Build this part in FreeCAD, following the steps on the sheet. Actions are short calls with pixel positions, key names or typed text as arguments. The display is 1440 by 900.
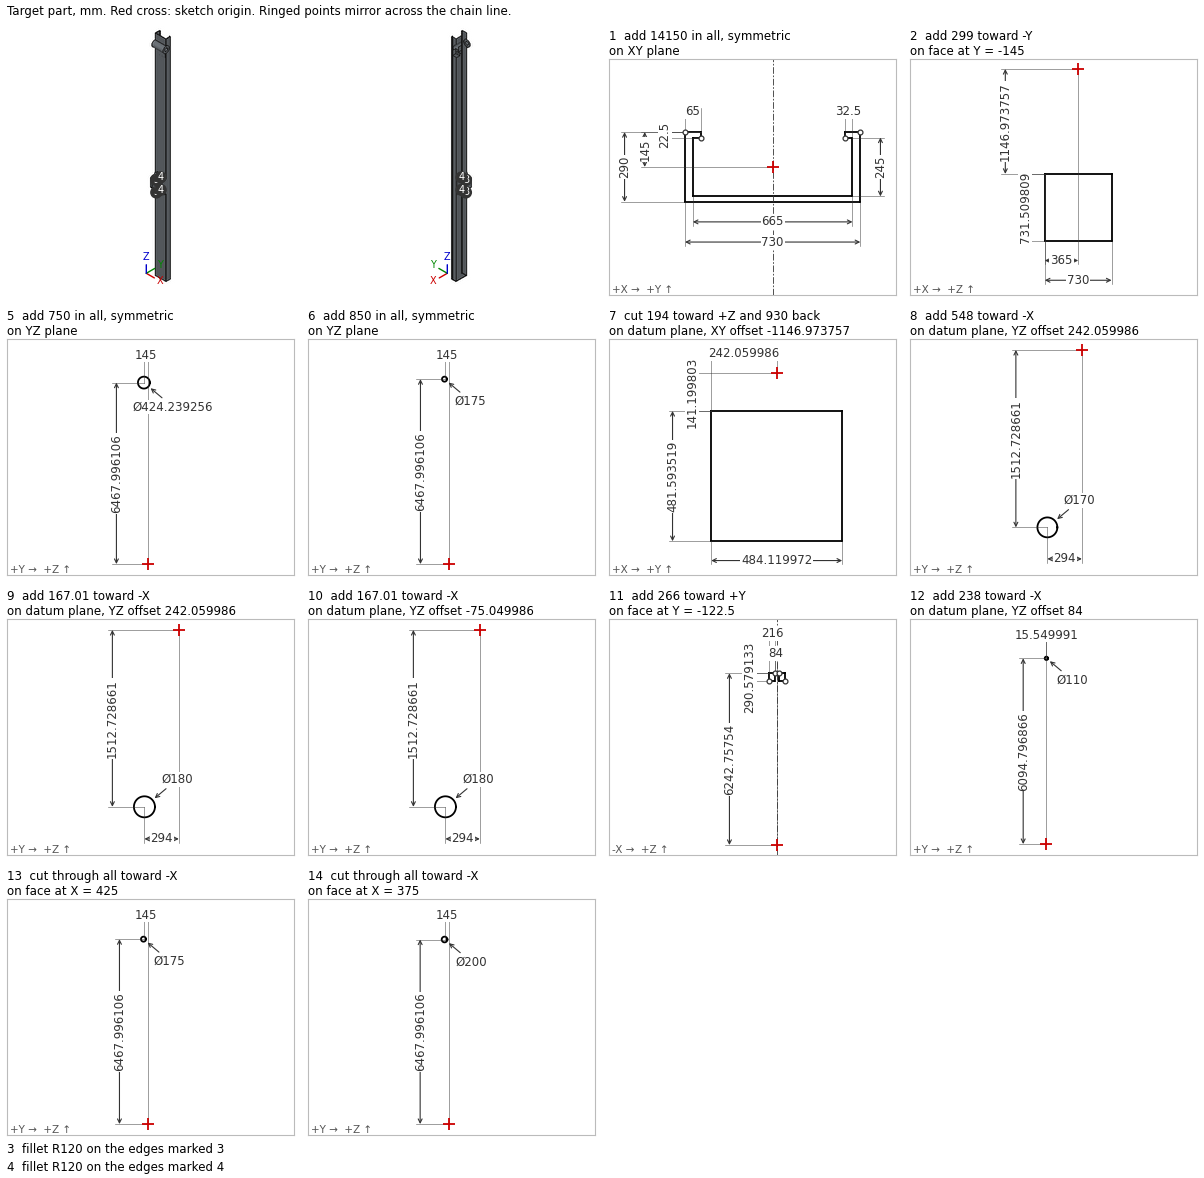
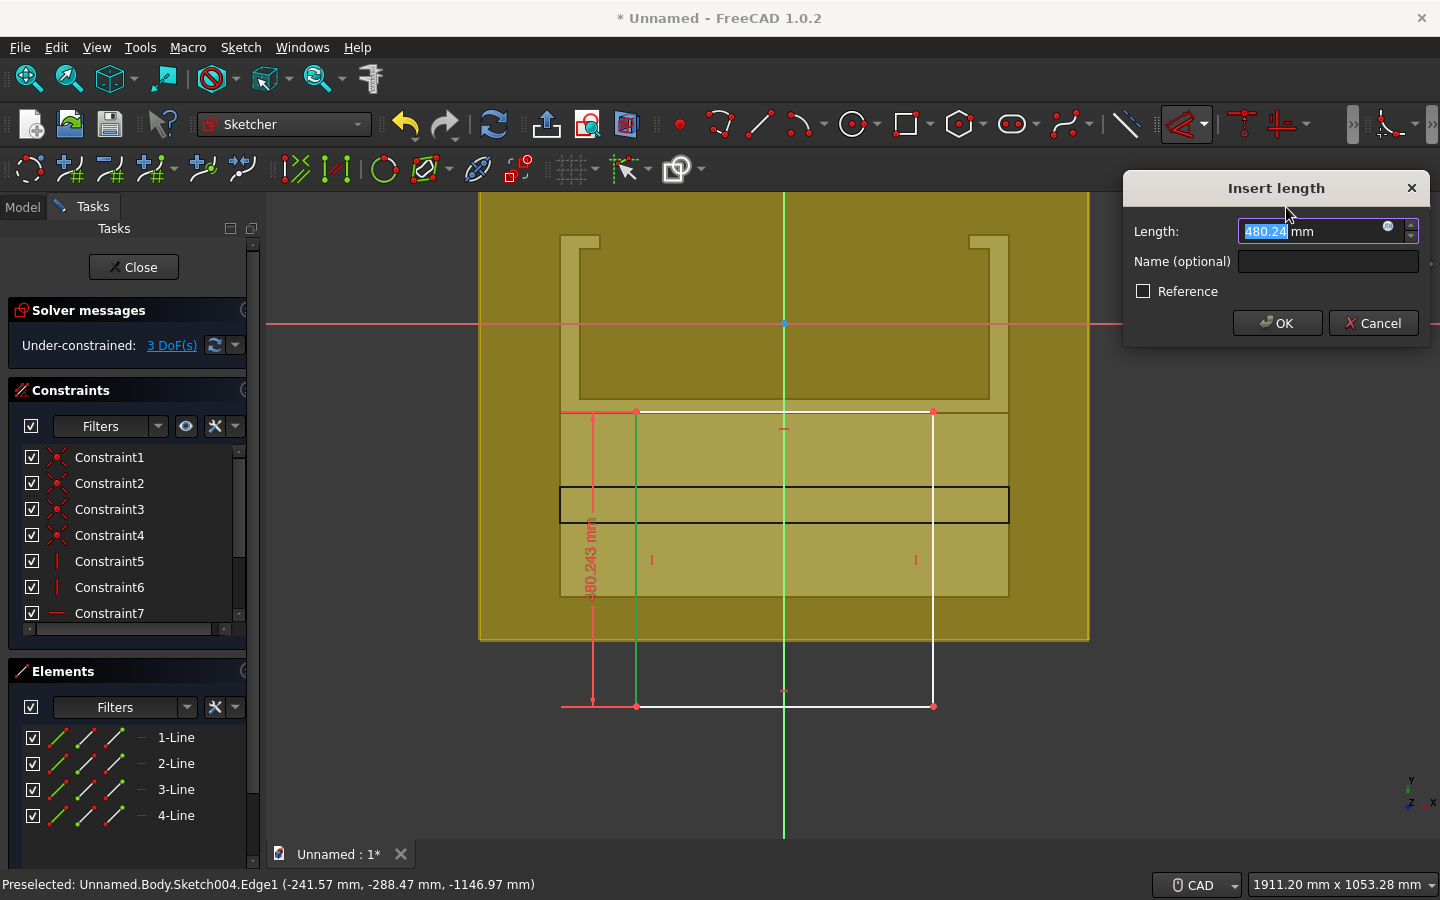
text(481.593519)
key(Return)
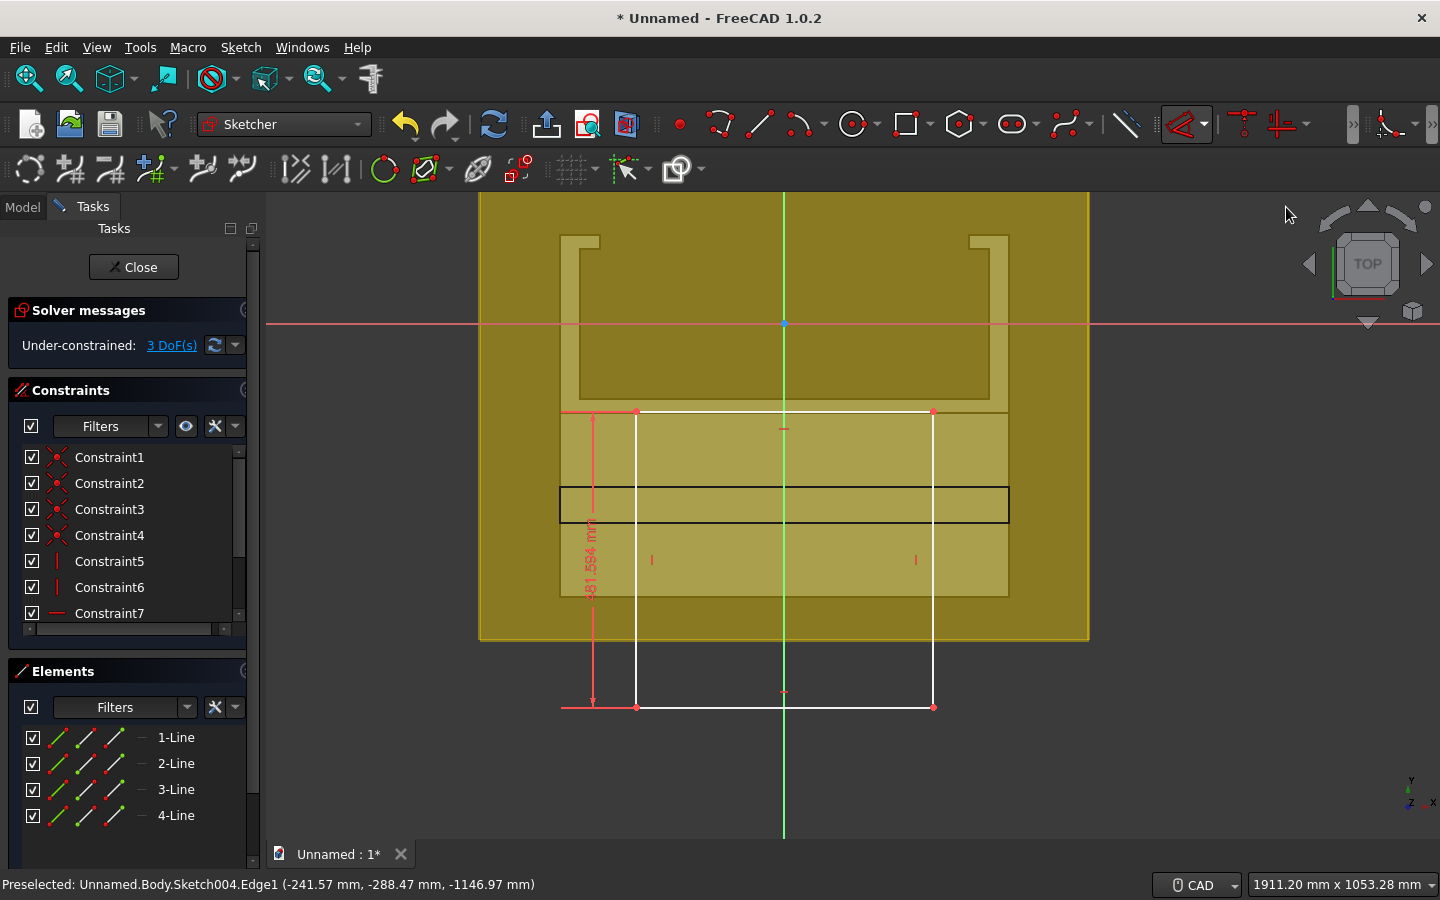
click(725, 708)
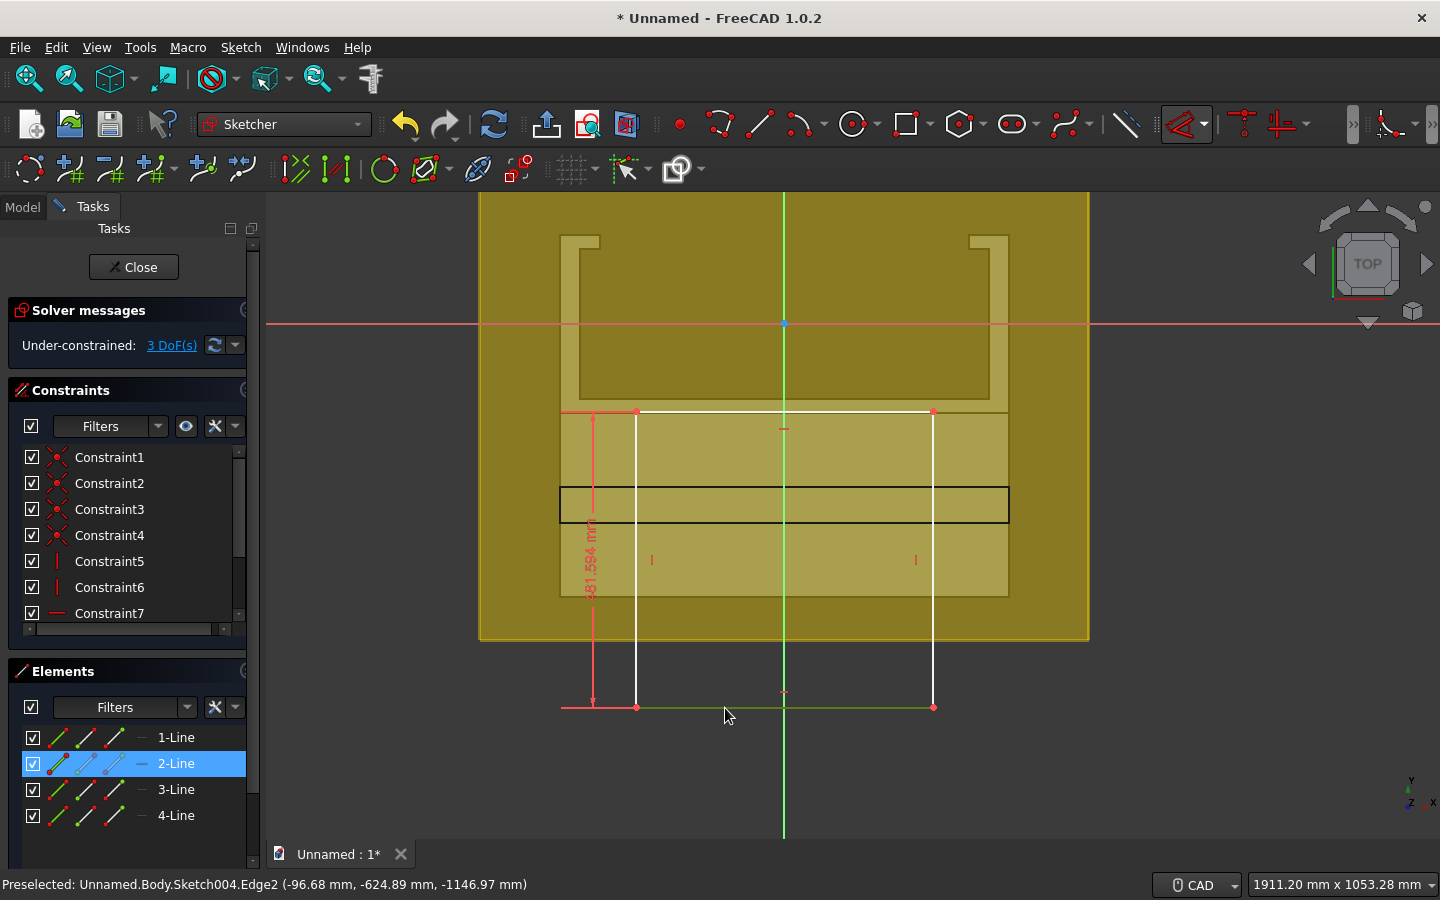
key(l)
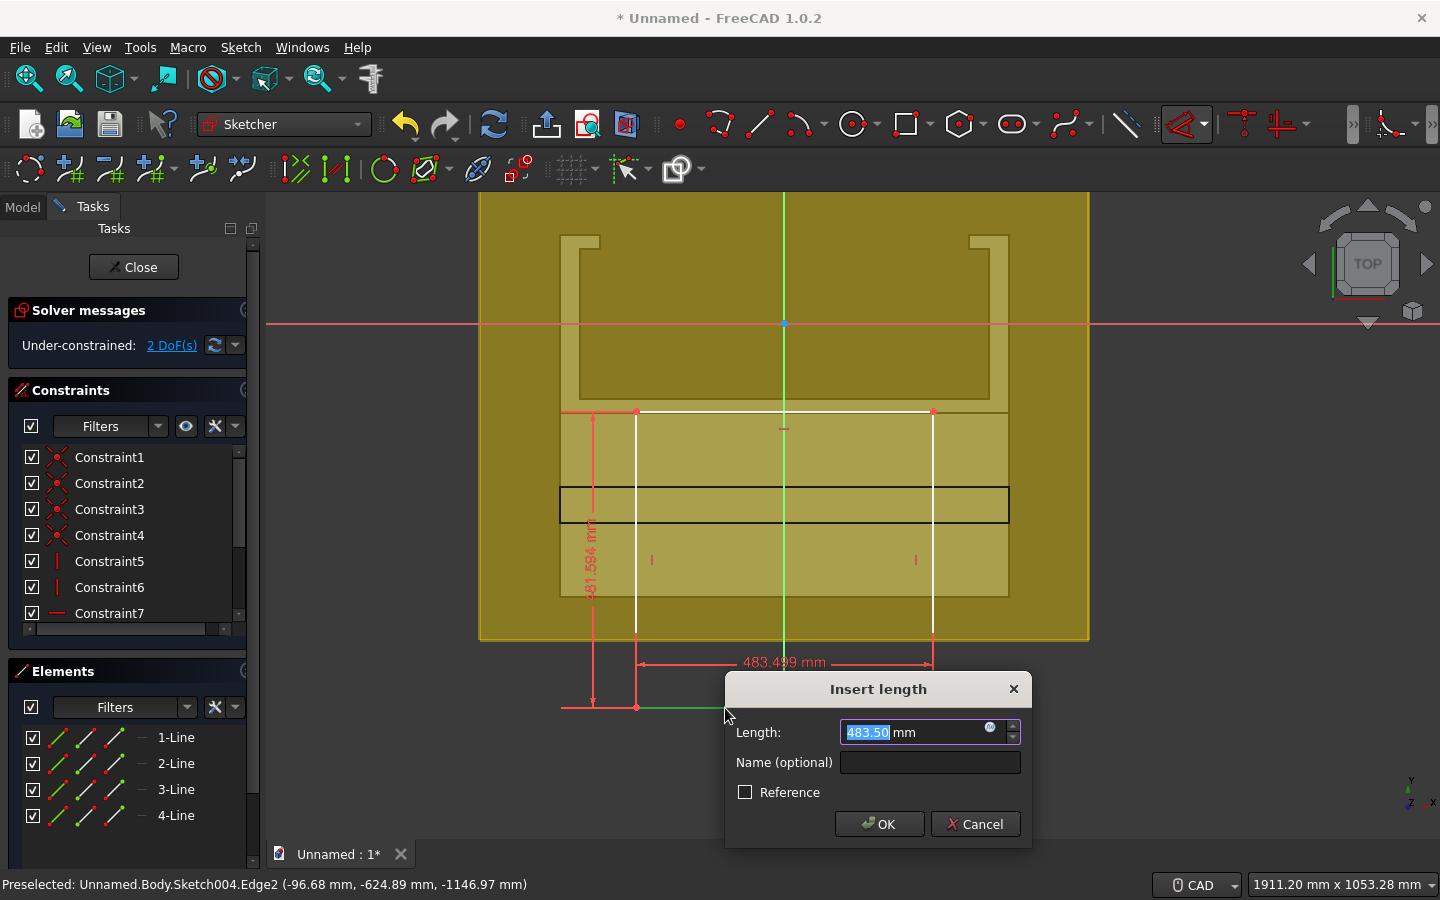
text(484.119972)
key(Return)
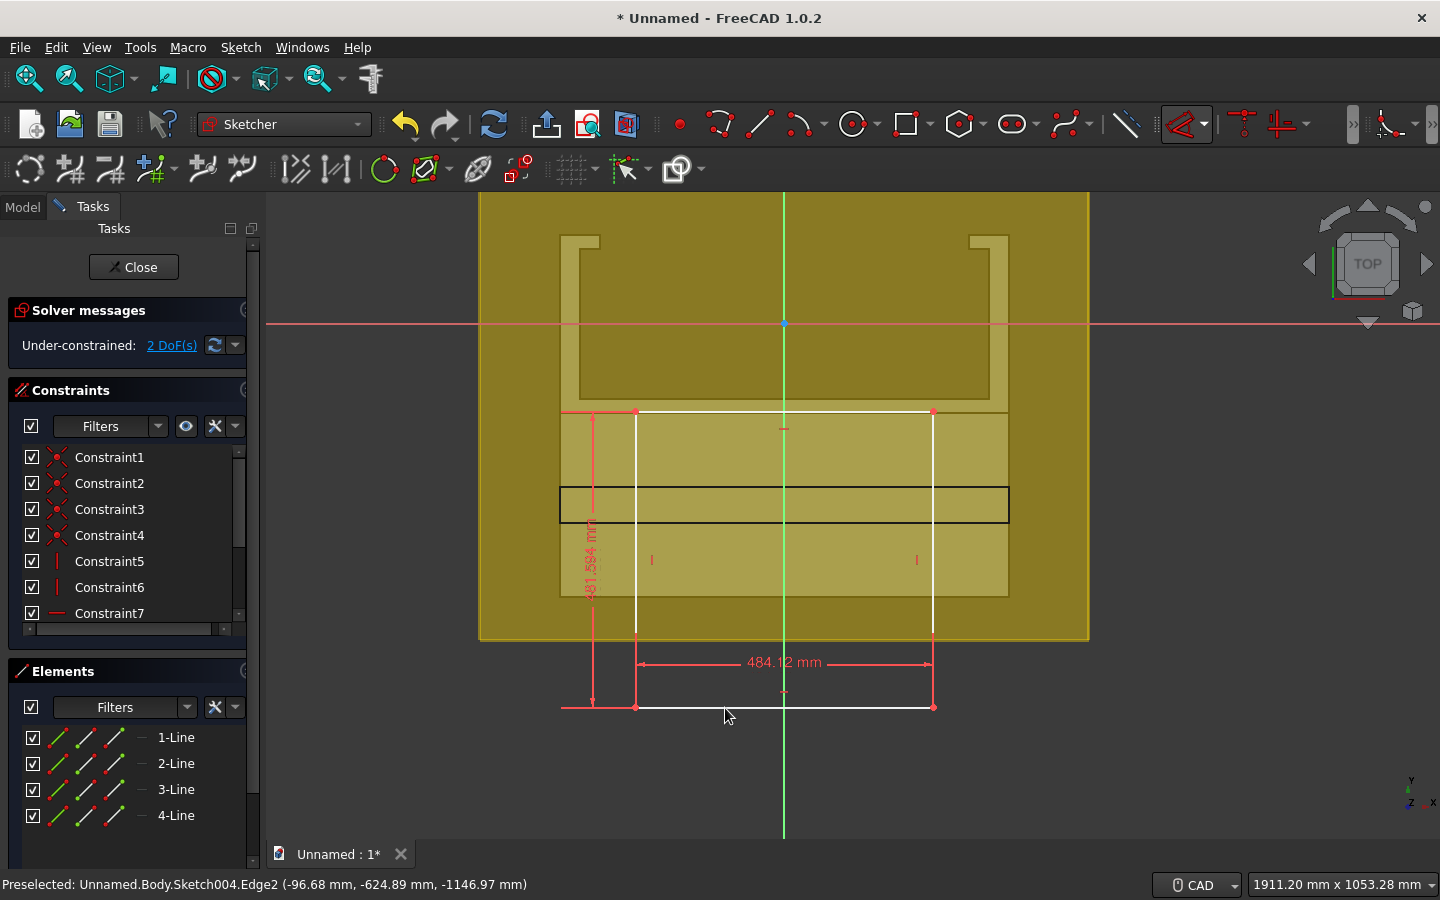
click(636, 412)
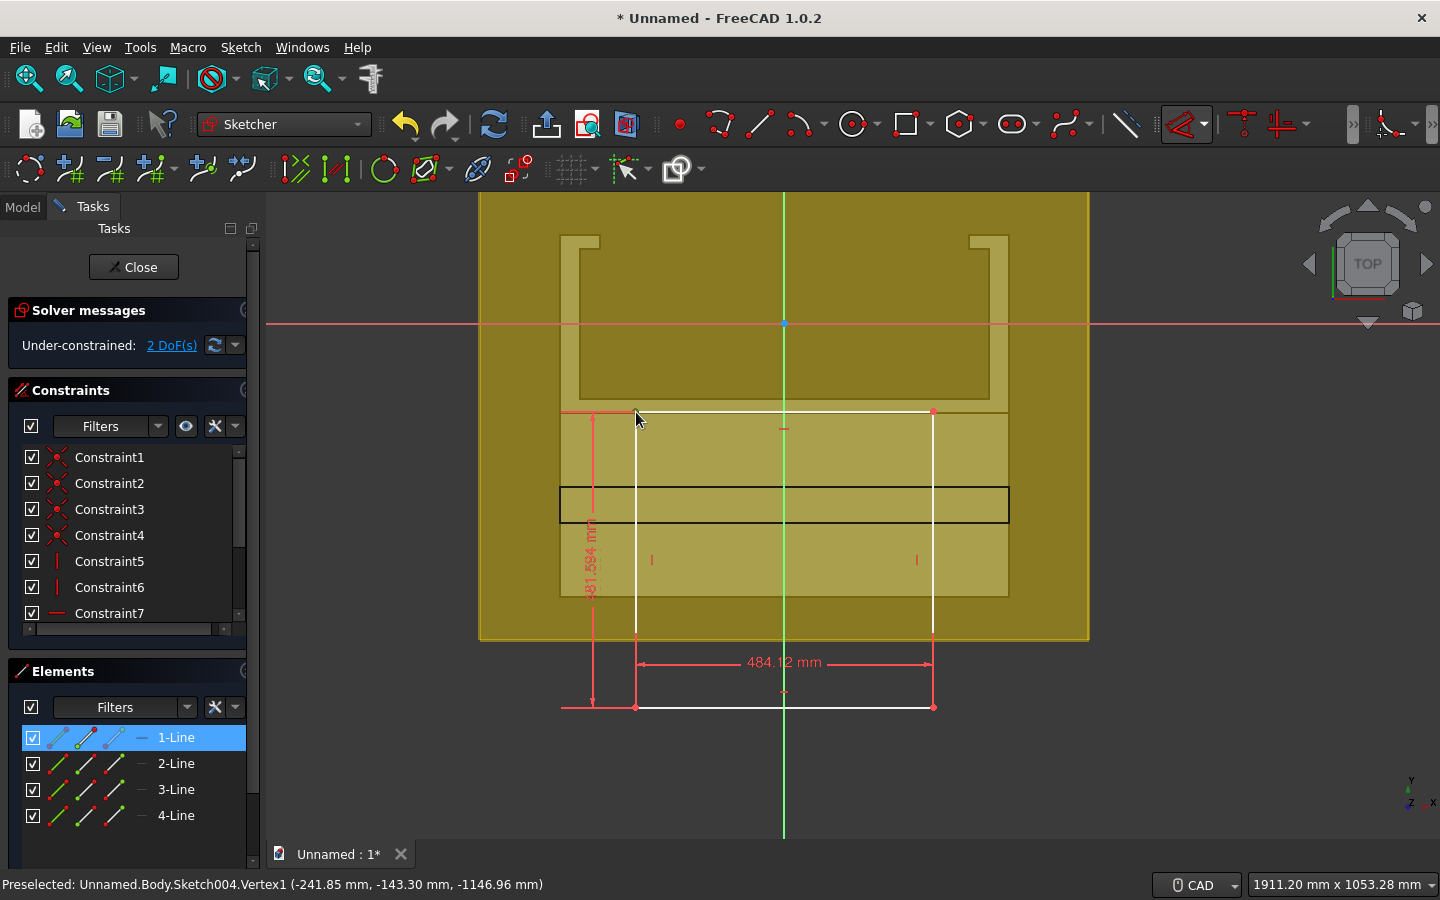
key(l)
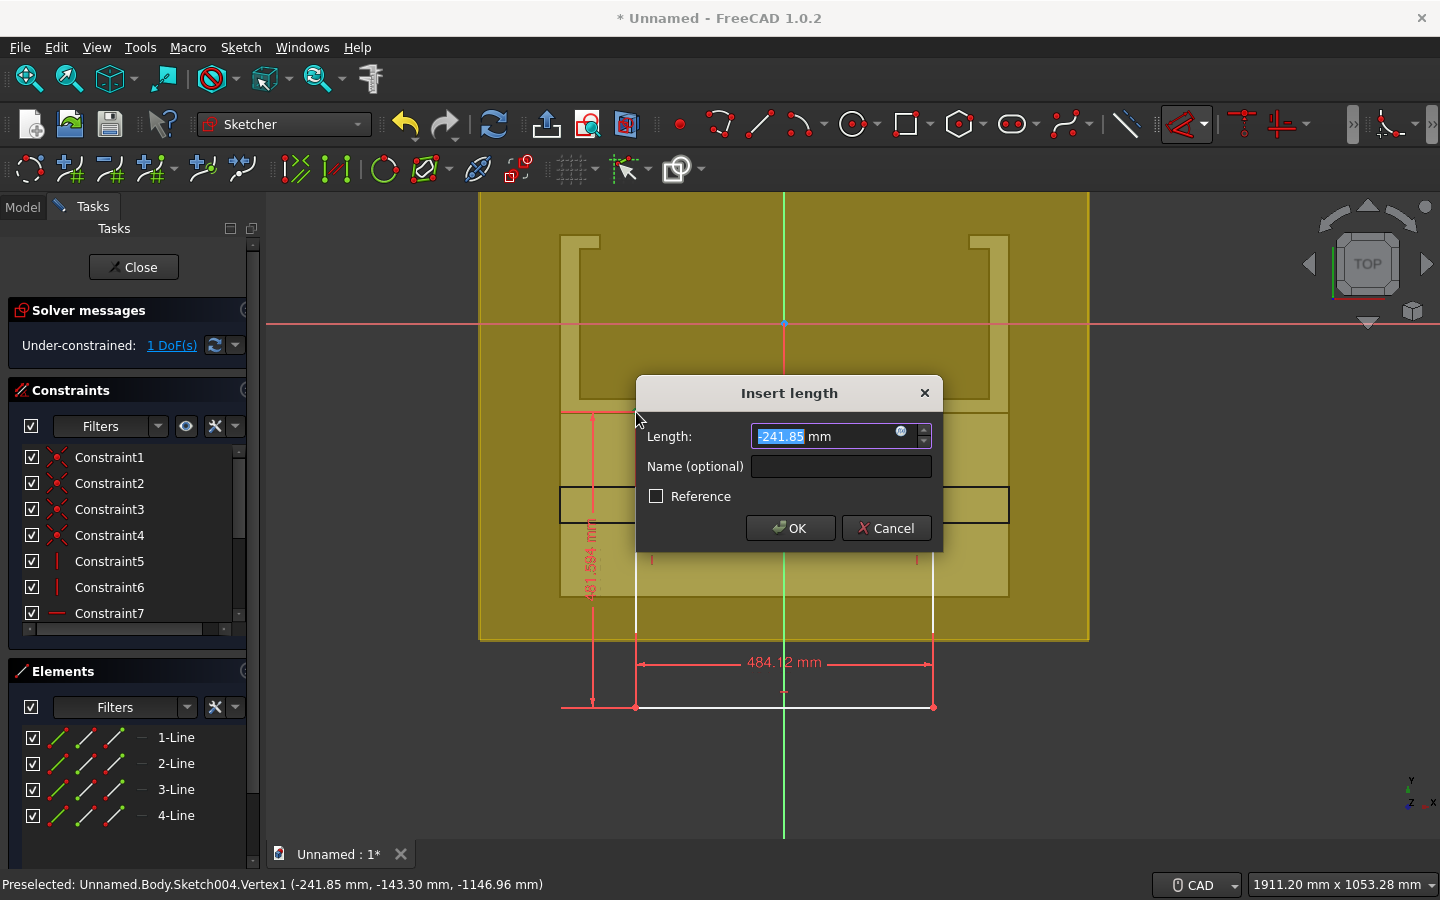
text(-242.059986)
key(Return)